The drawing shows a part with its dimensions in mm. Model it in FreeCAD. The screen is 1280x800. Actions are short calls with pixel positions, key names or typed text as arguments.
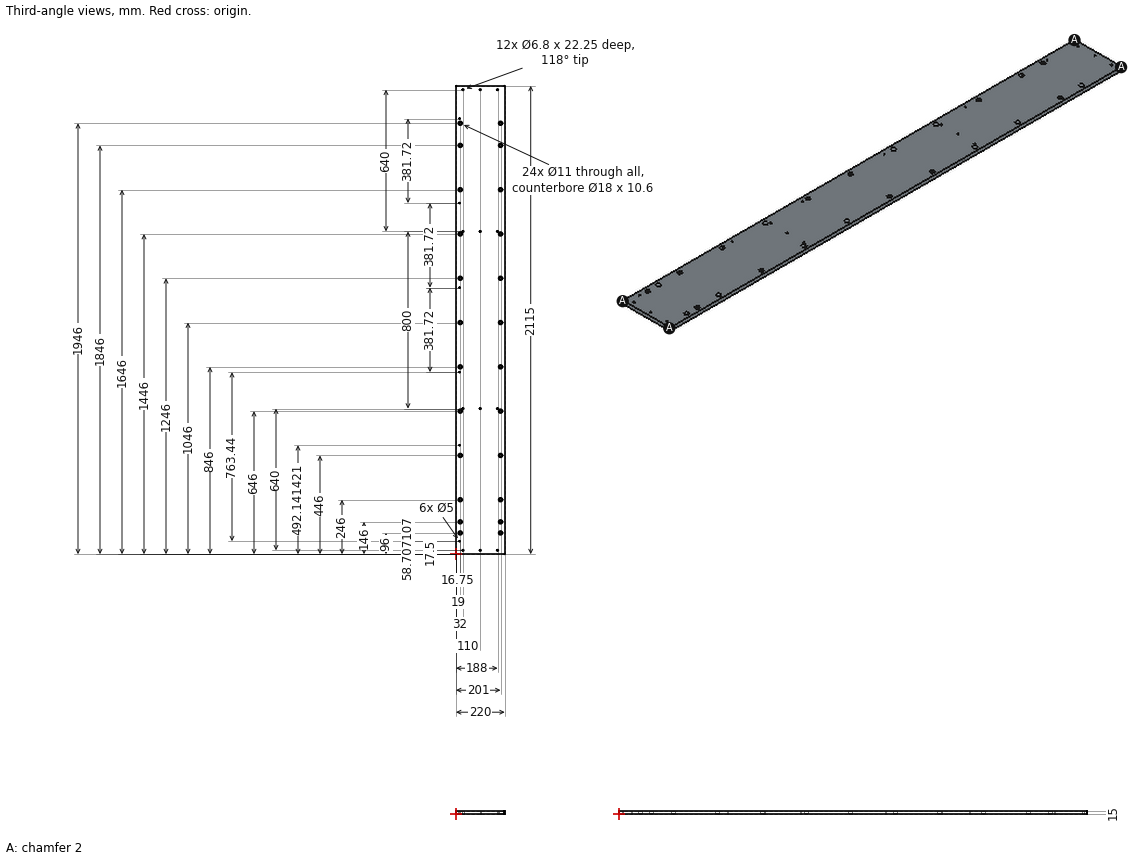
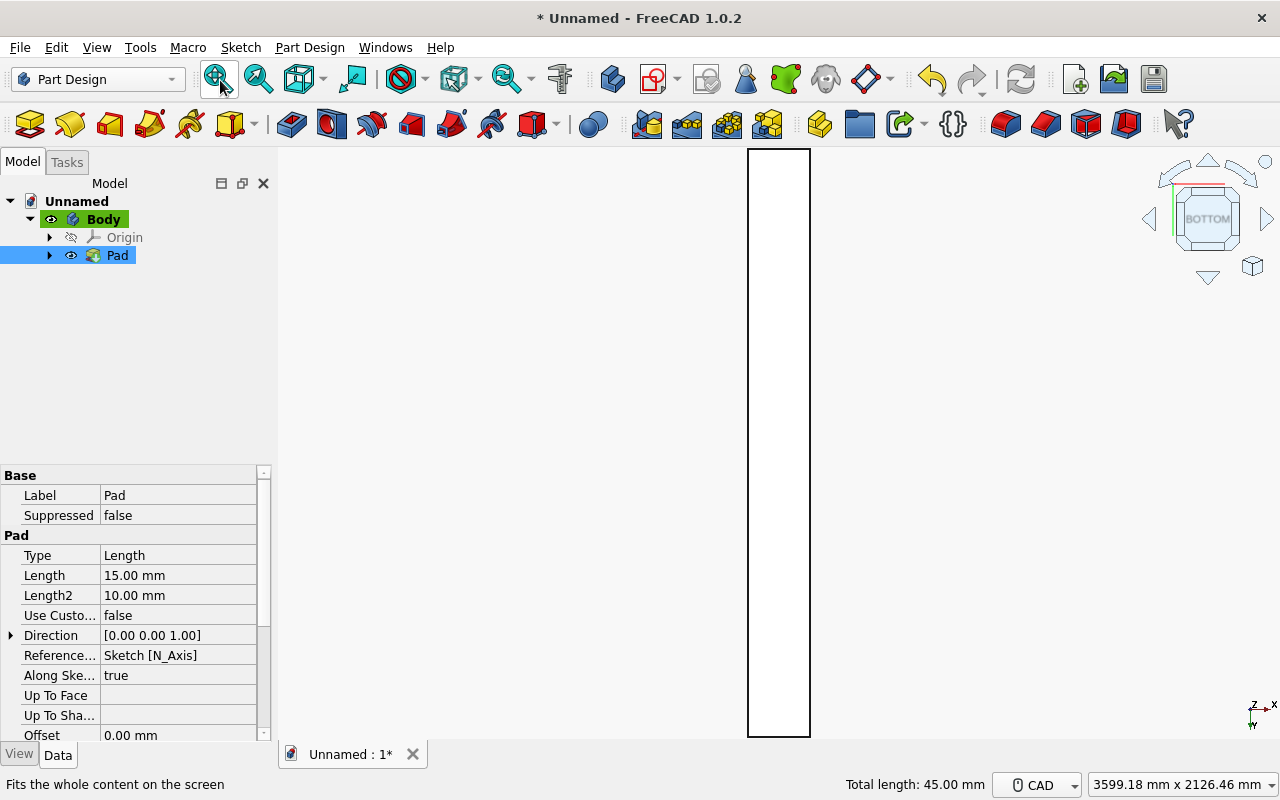
key(4)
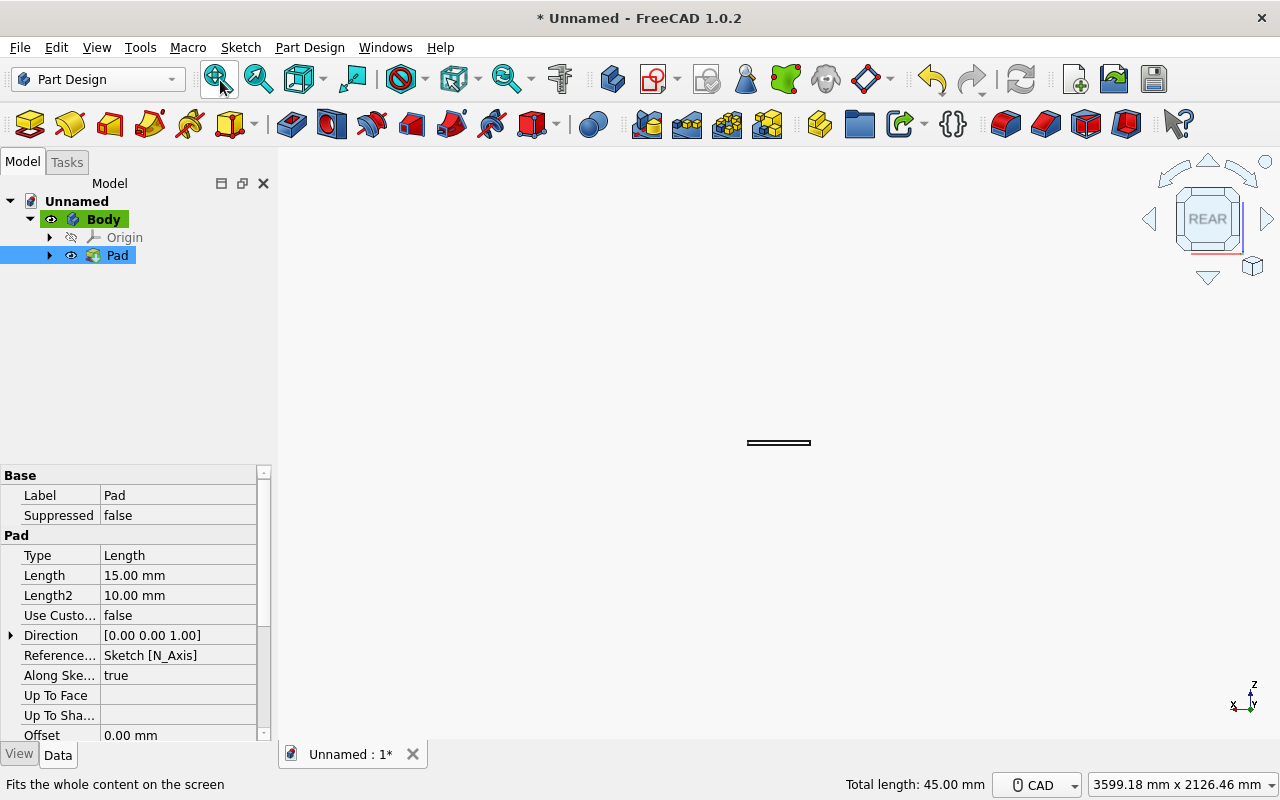
click(220, 80)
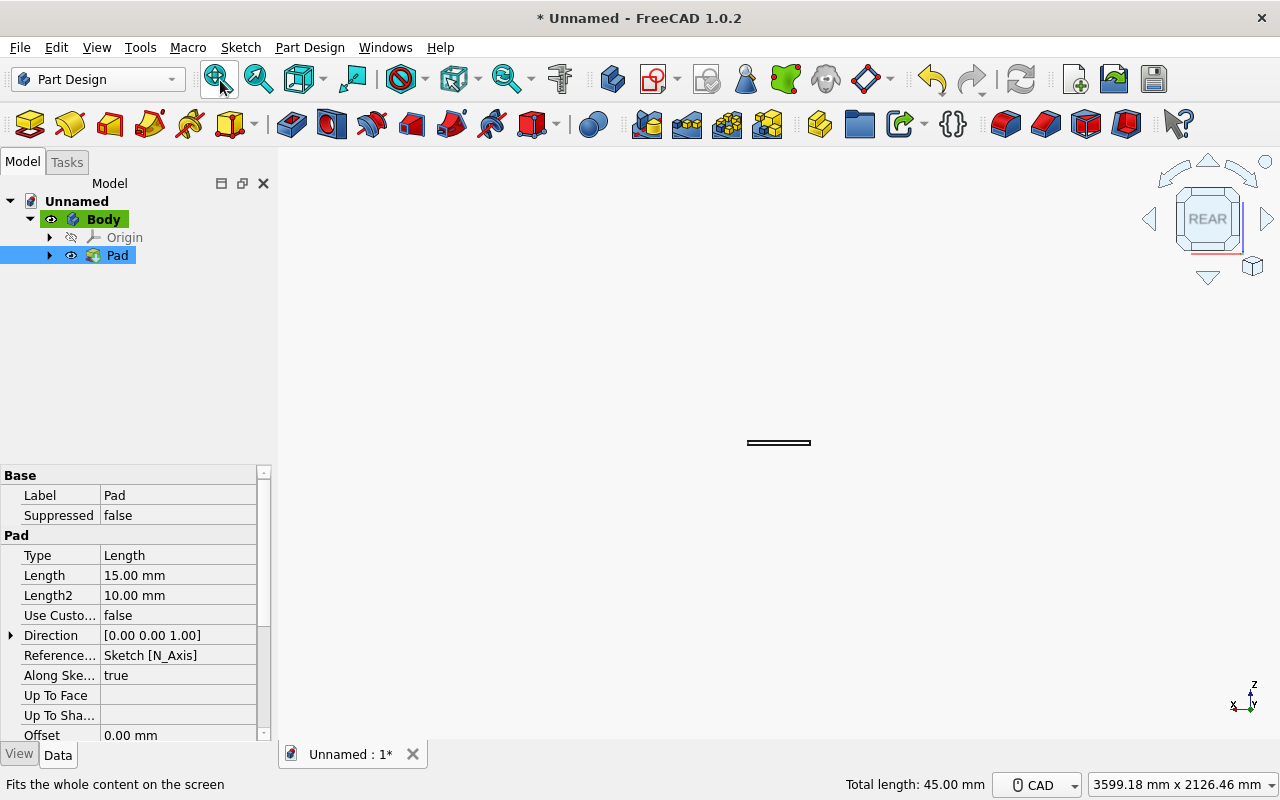
scroll(810, 442, up, 12)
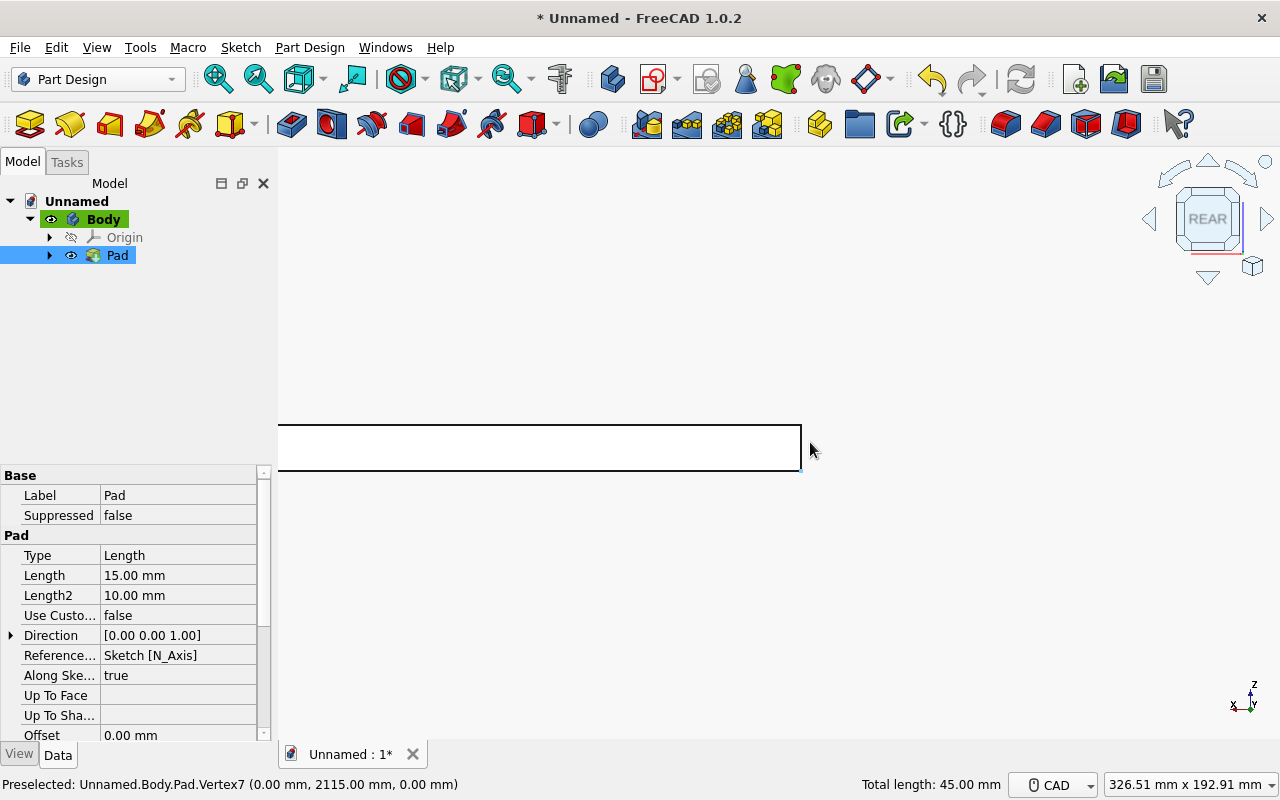
click(801, 447, ctrl)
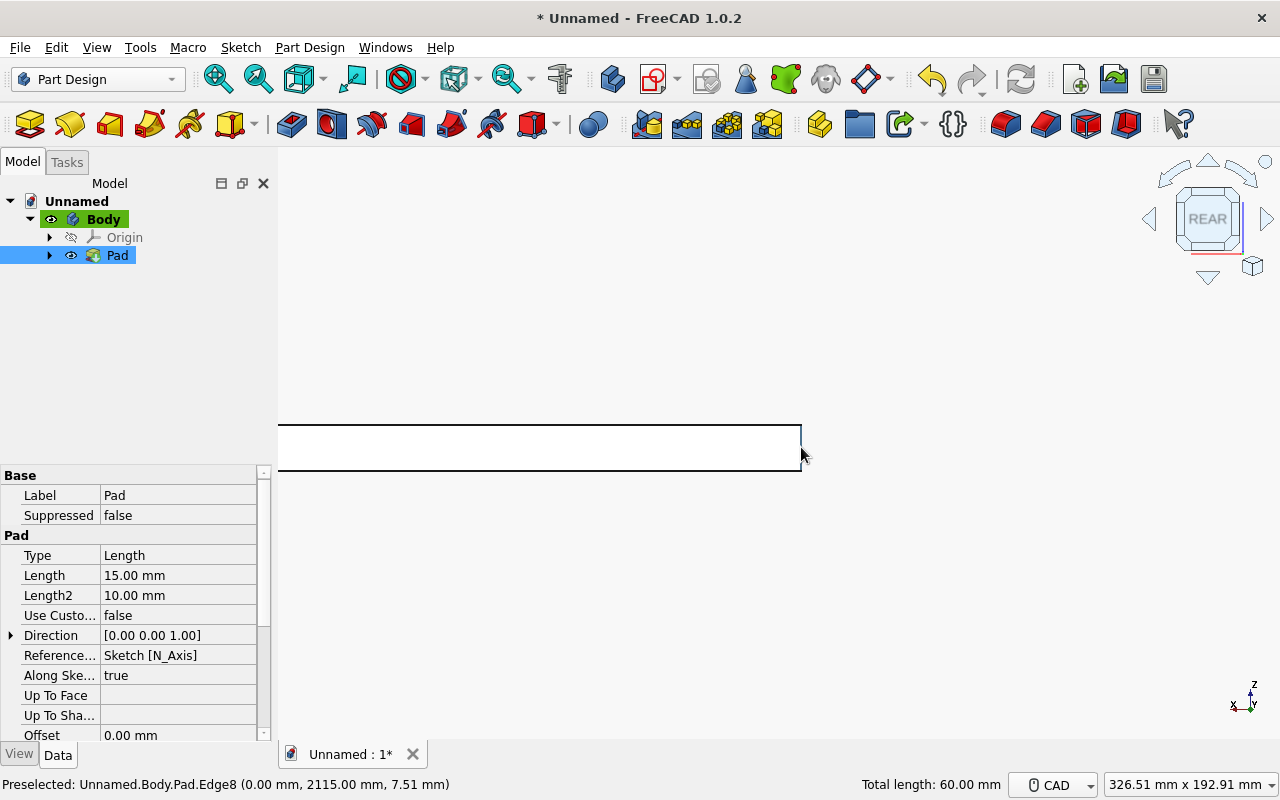
click(1046, 124)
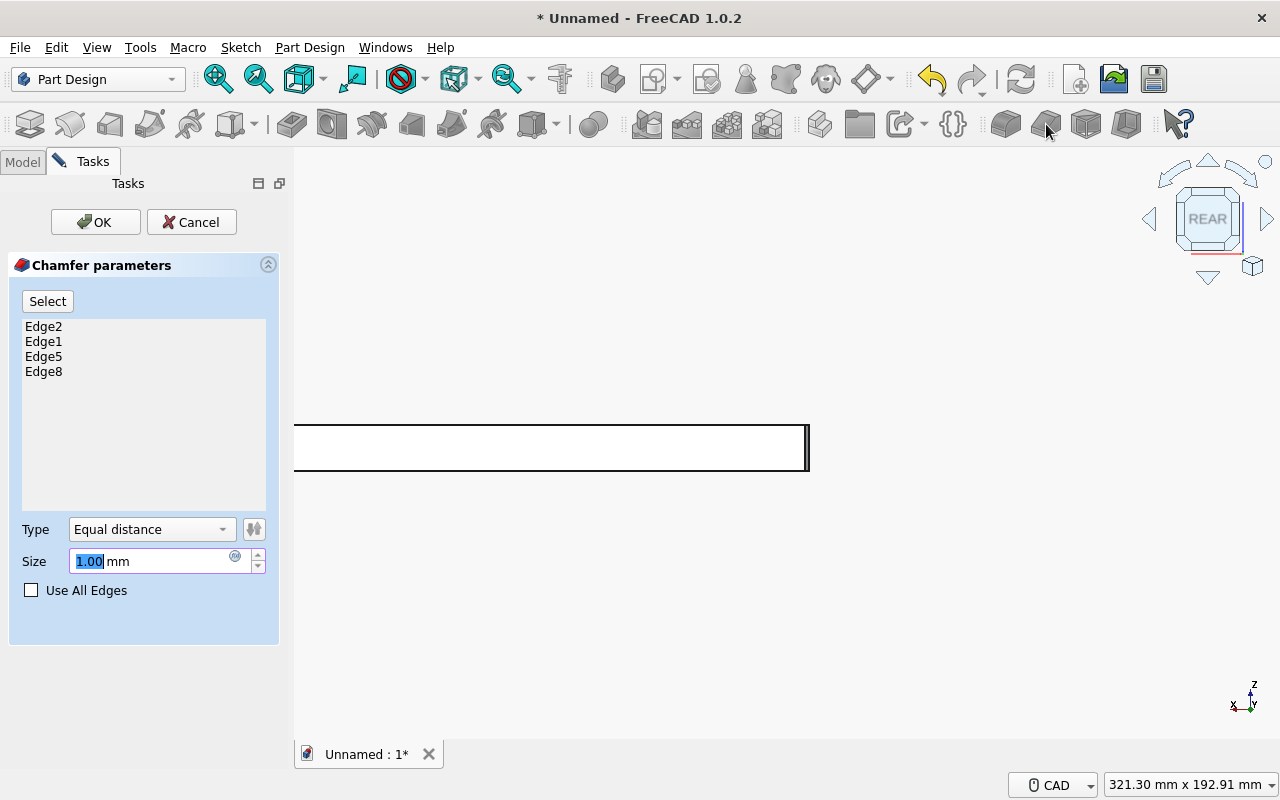
text(2)
key(Tab)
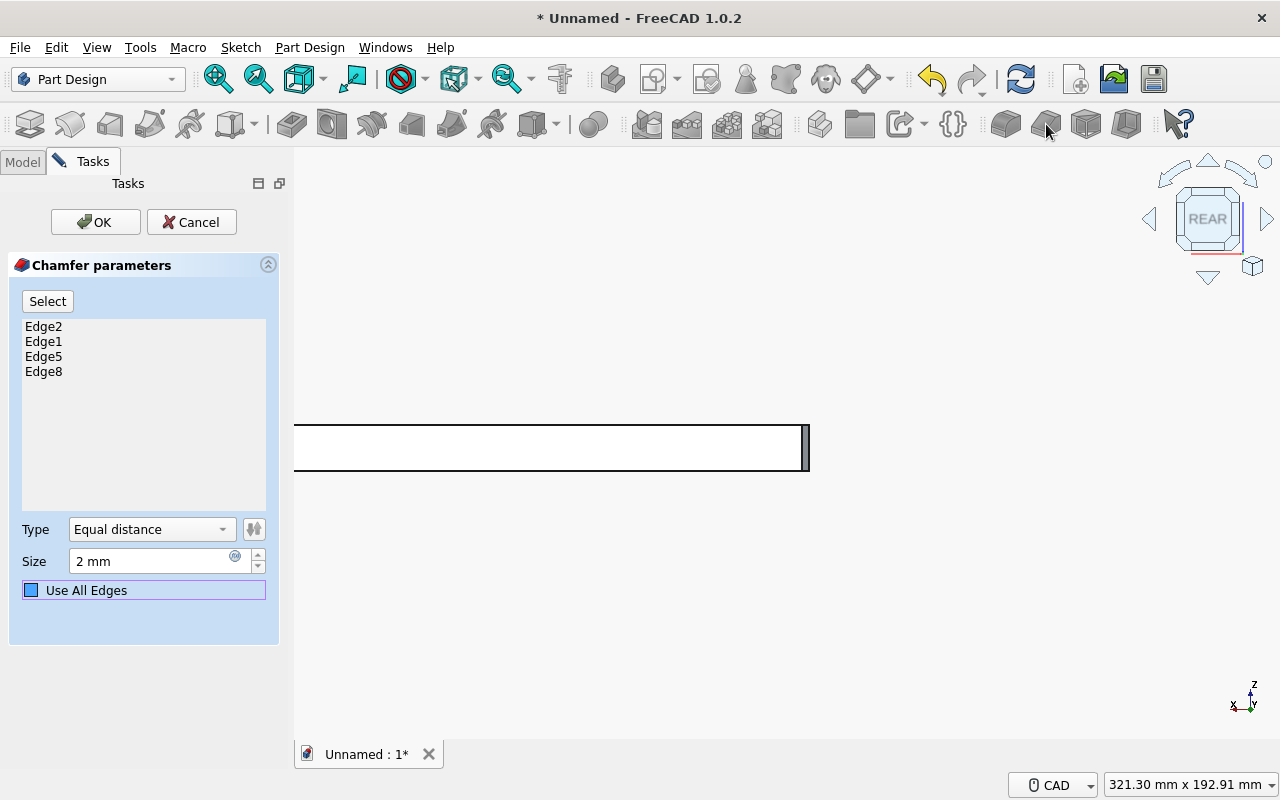
click(96, 222)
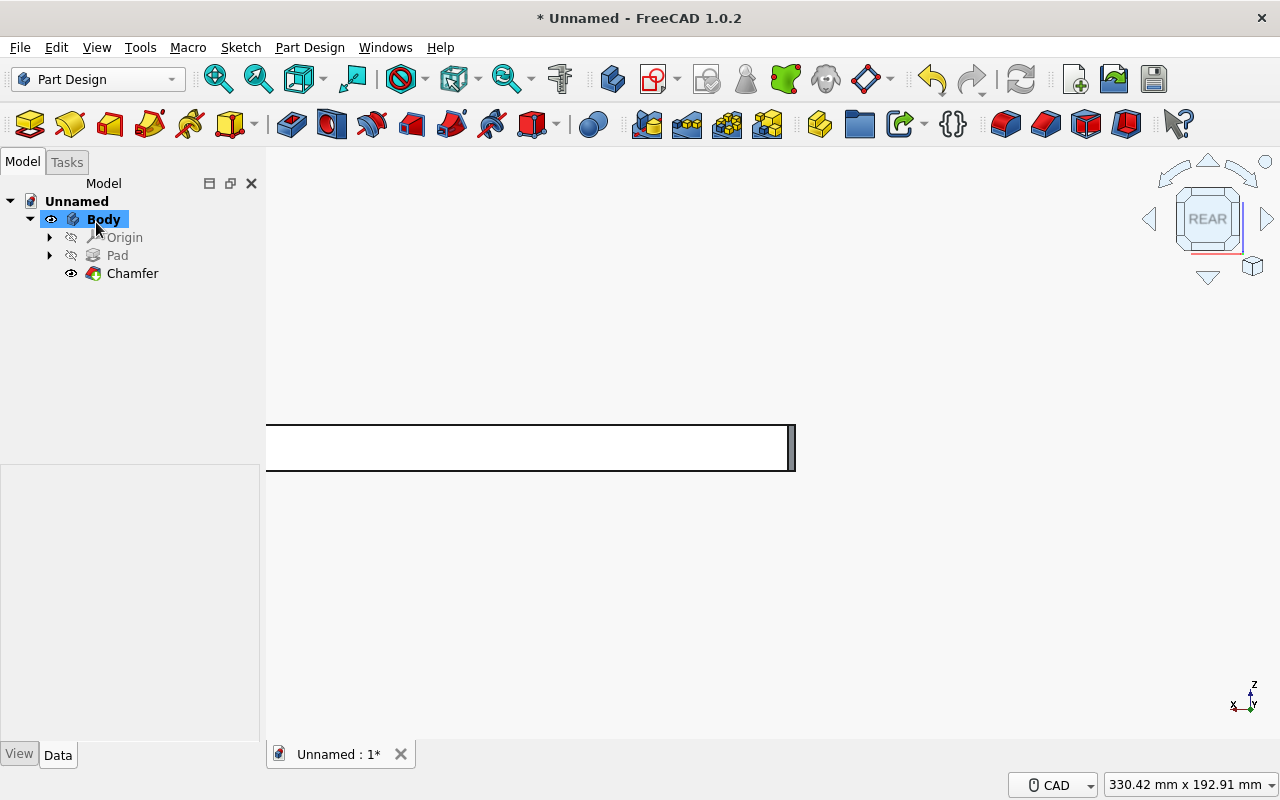
click(220, 80)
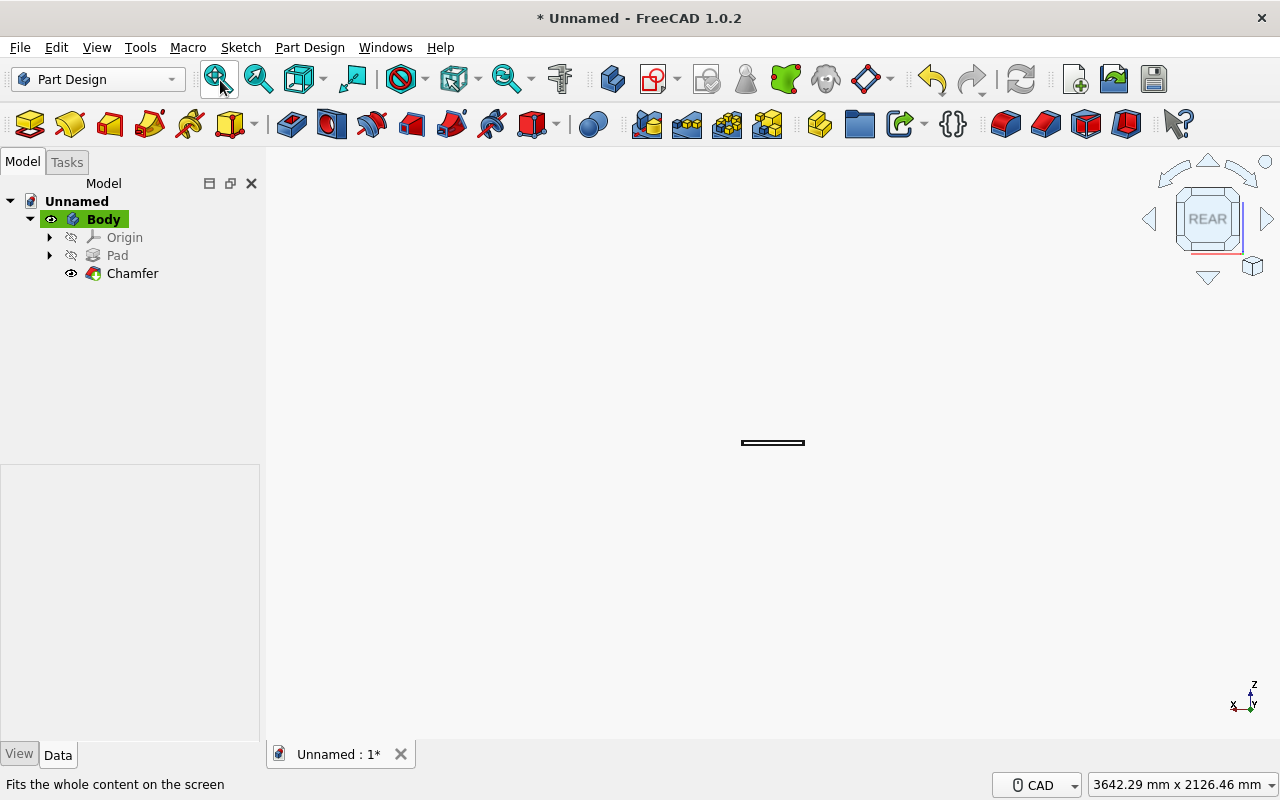
key(0)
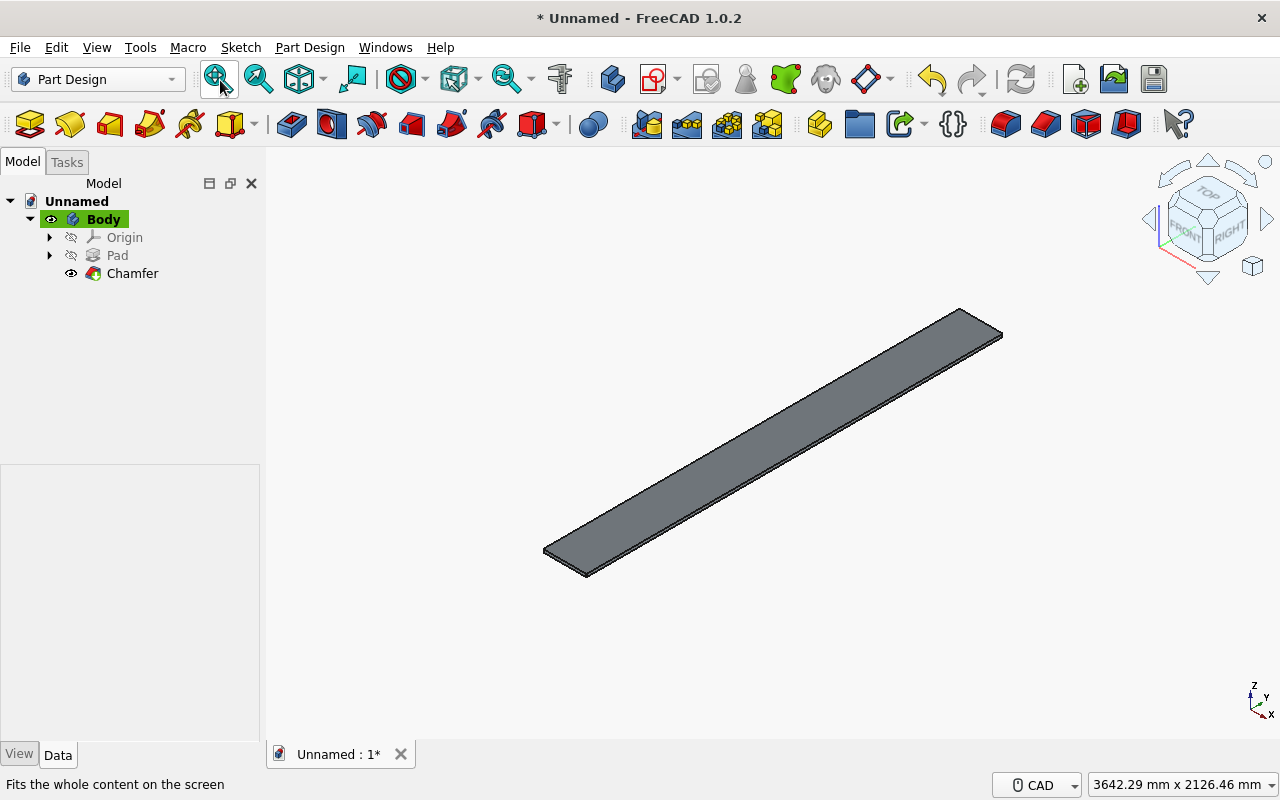
click(951, 337)